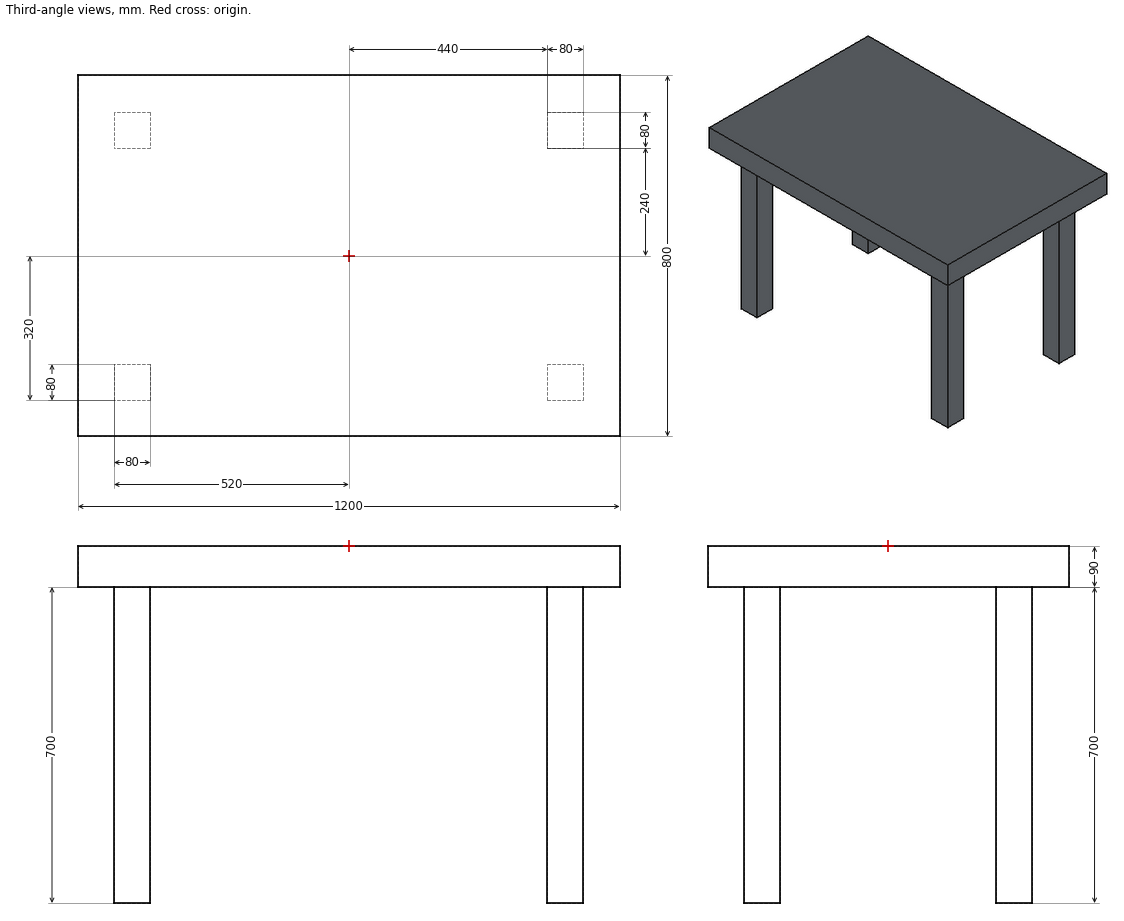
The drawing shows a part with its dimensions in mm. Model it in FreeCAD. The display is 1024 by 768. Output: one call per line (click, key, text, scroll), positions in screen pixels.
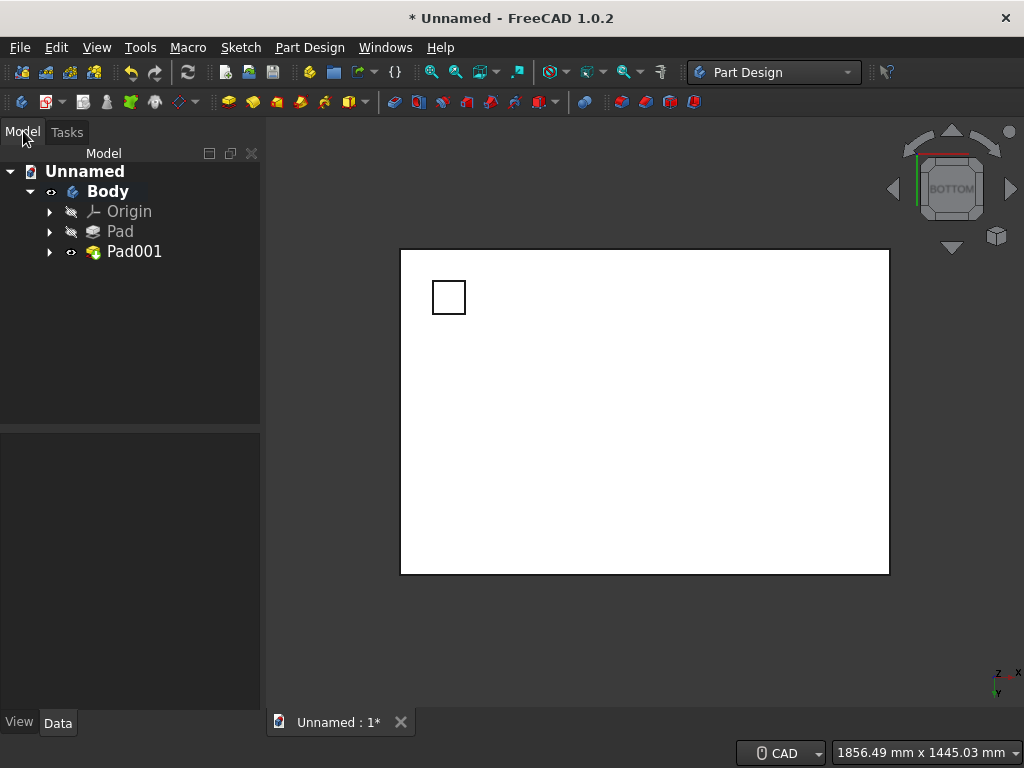
click(116, 252)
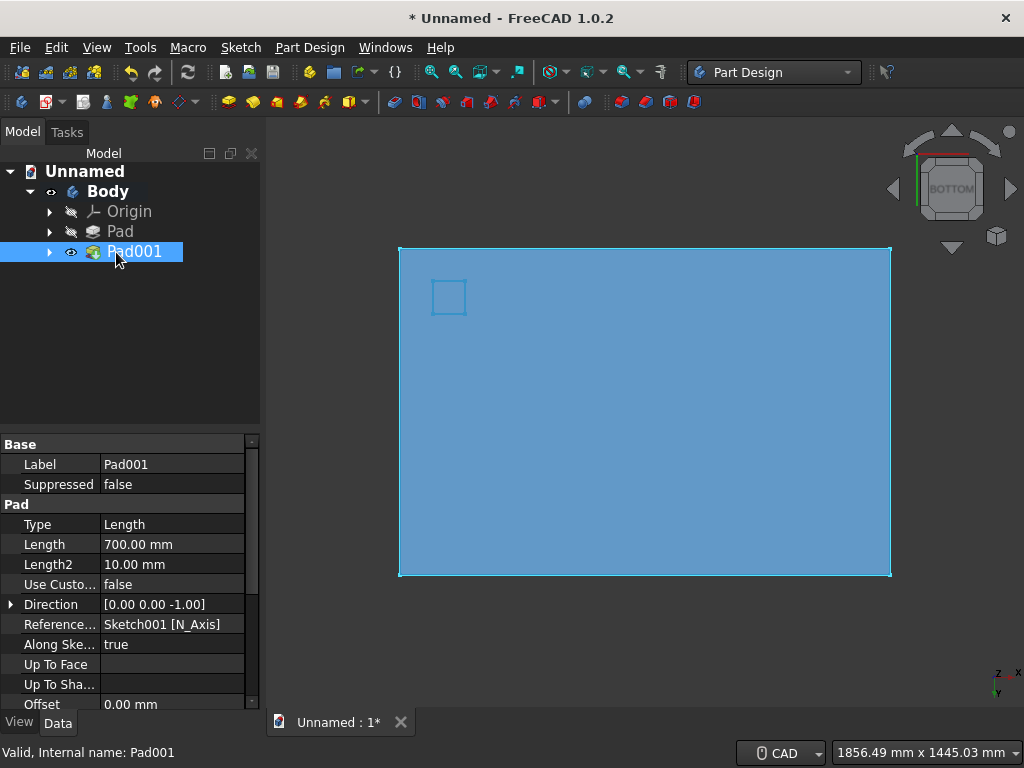
click(22, 72)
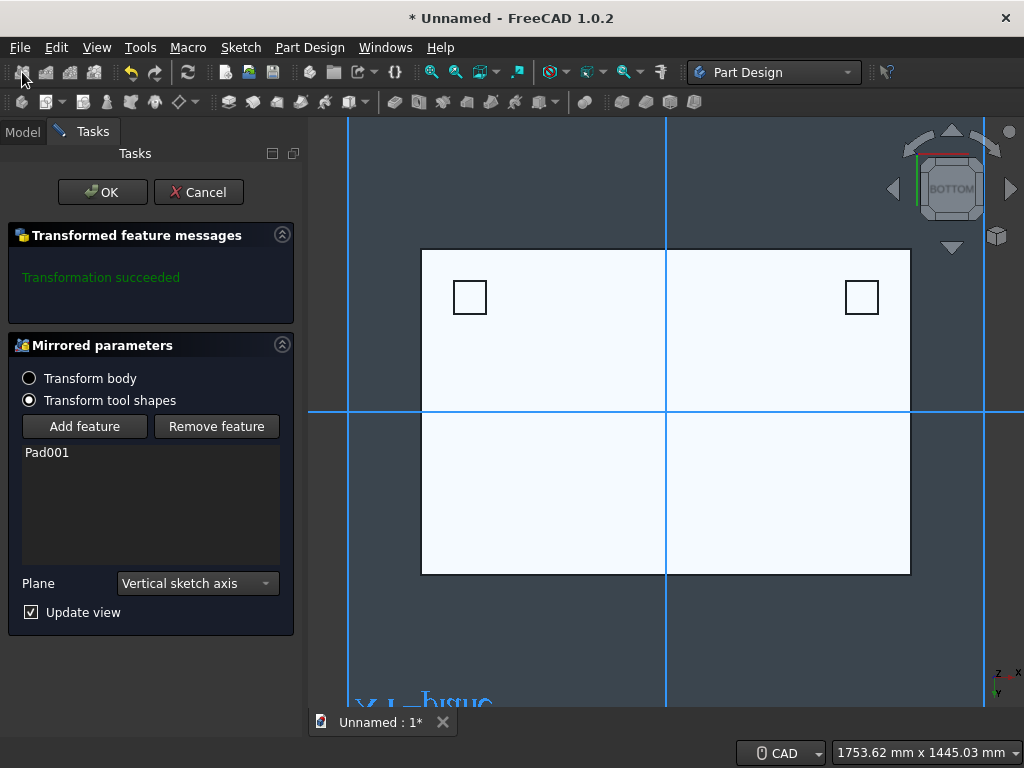
click(198, 584)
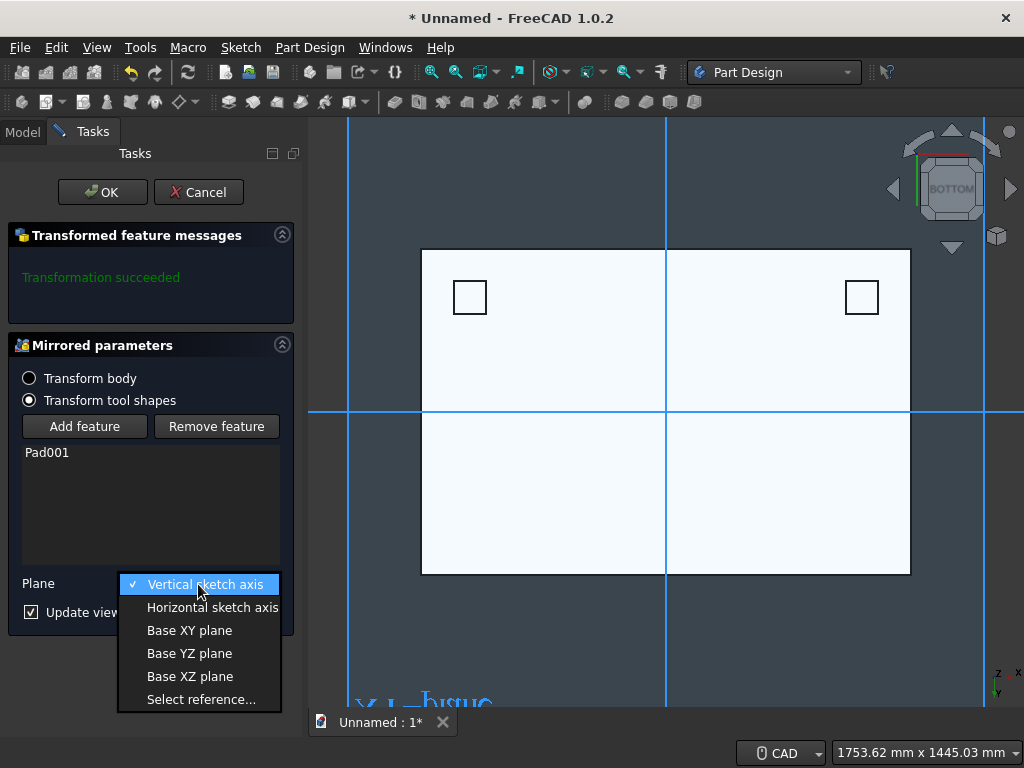
click(198, 676)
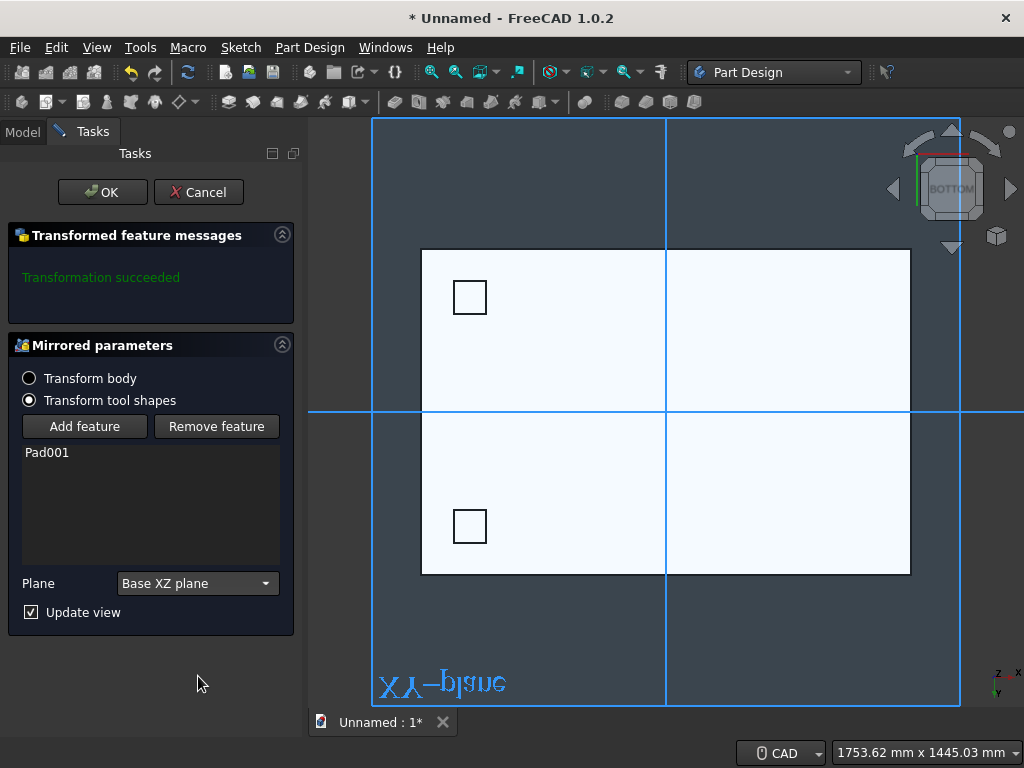
click(103, 192)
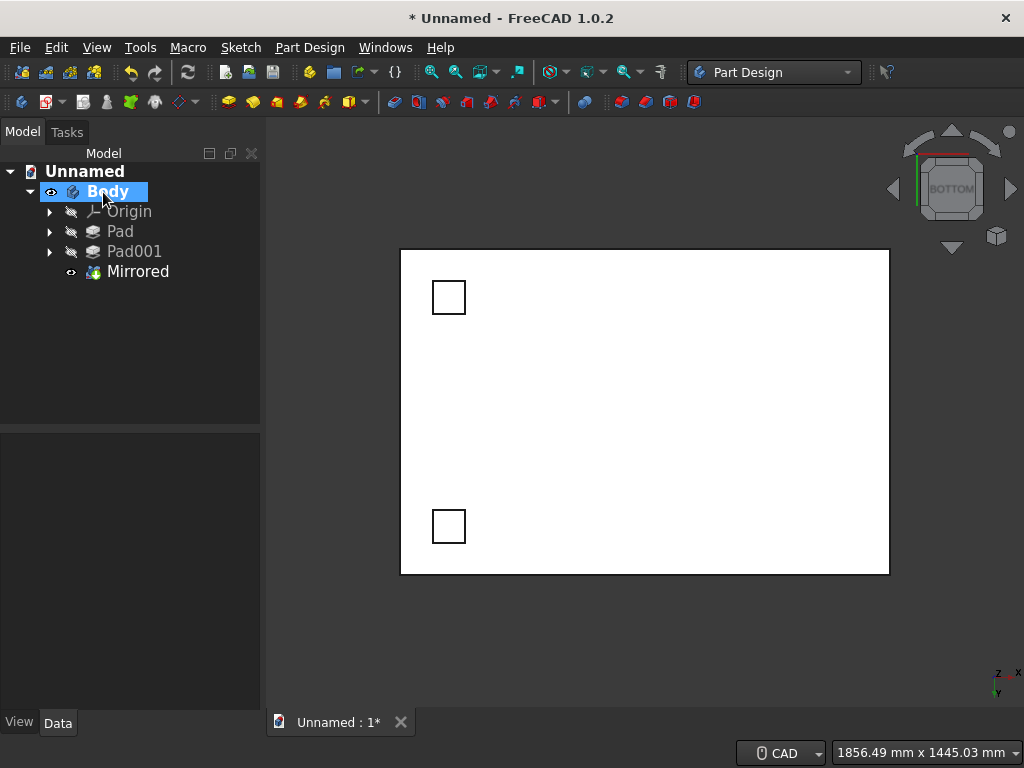
click(116, 252)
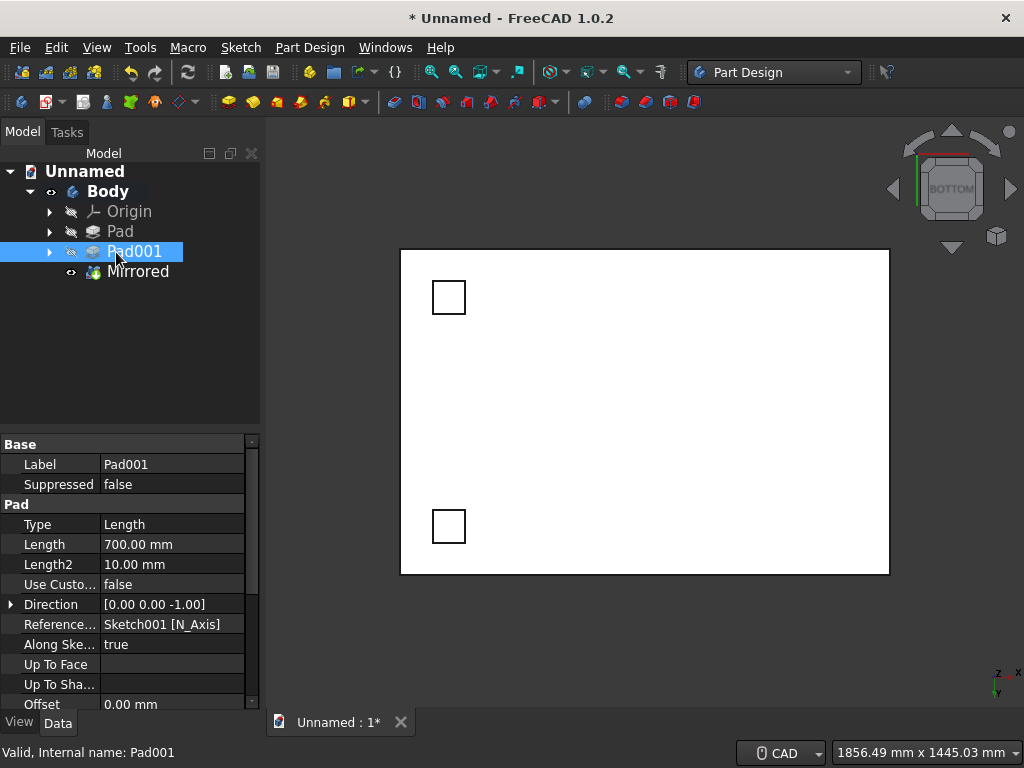
click(22, 72)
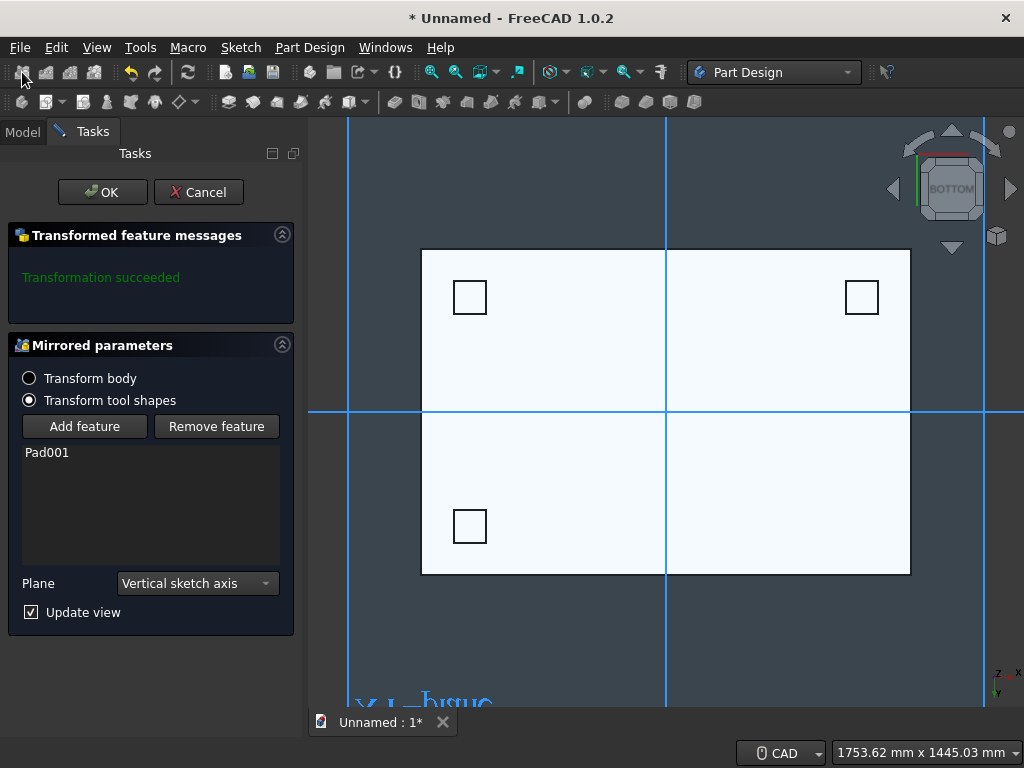
click(198, 584)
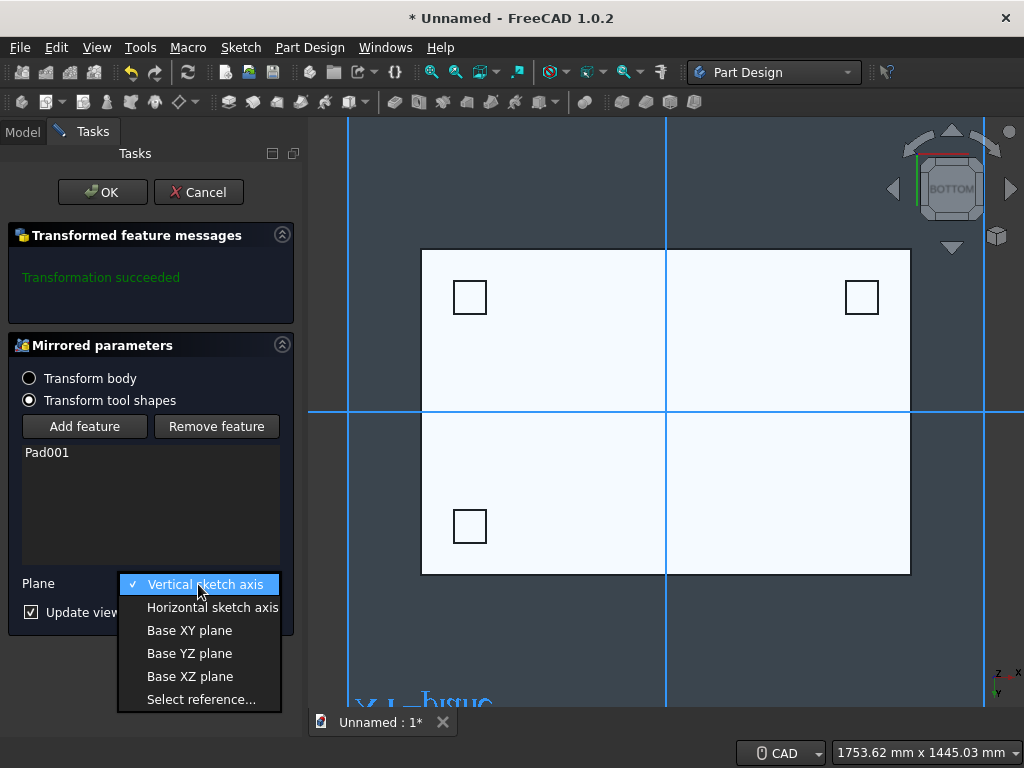
click(198, 654)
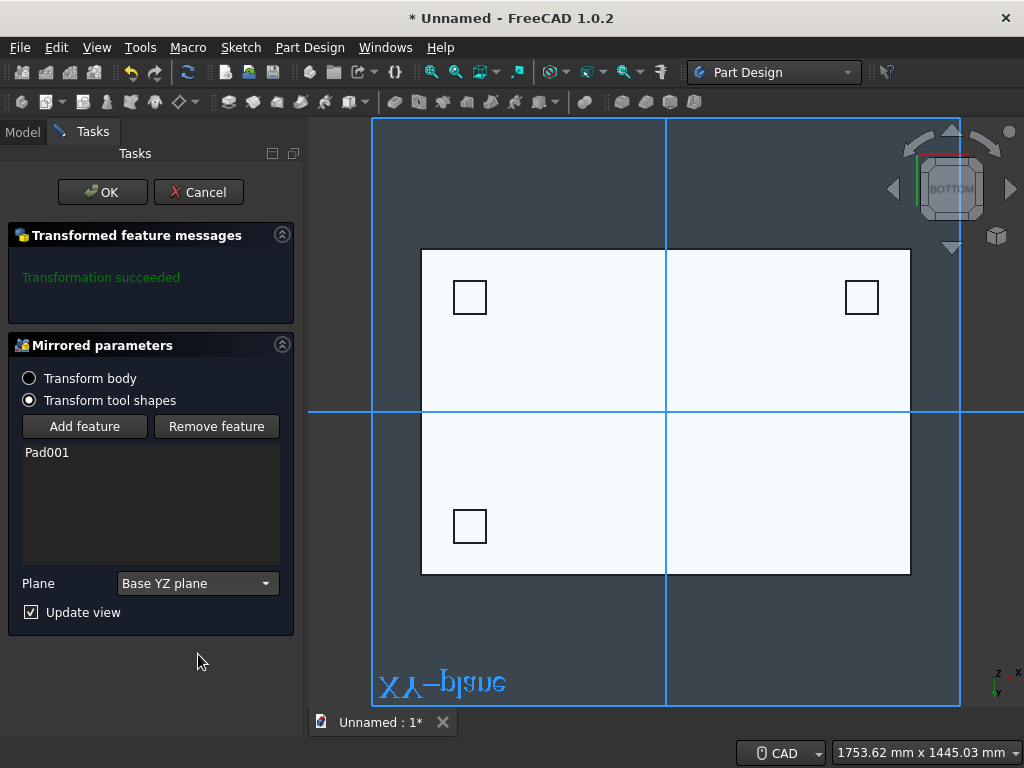
click(103, 192)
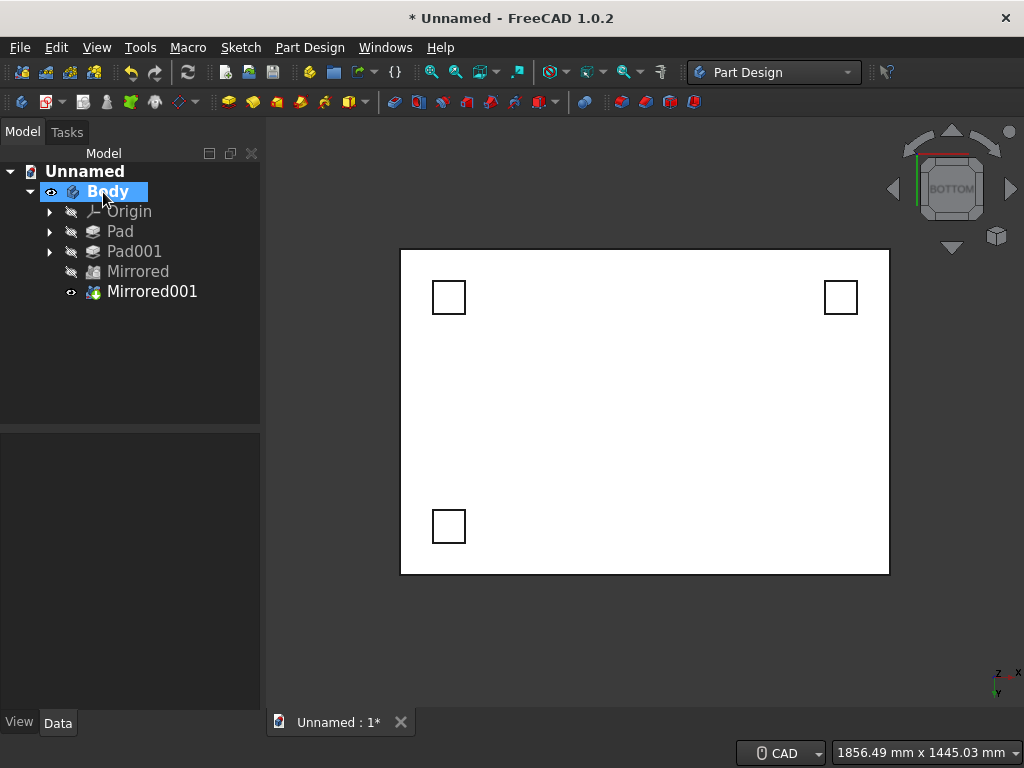
click(645, 411)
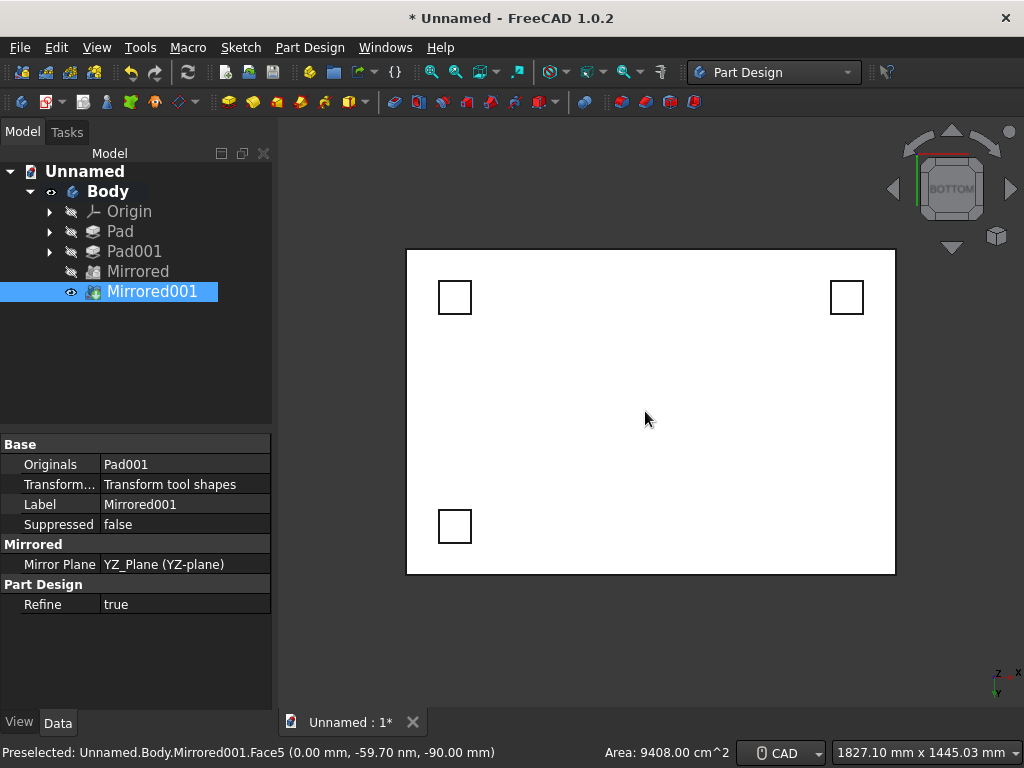
click(46, 102)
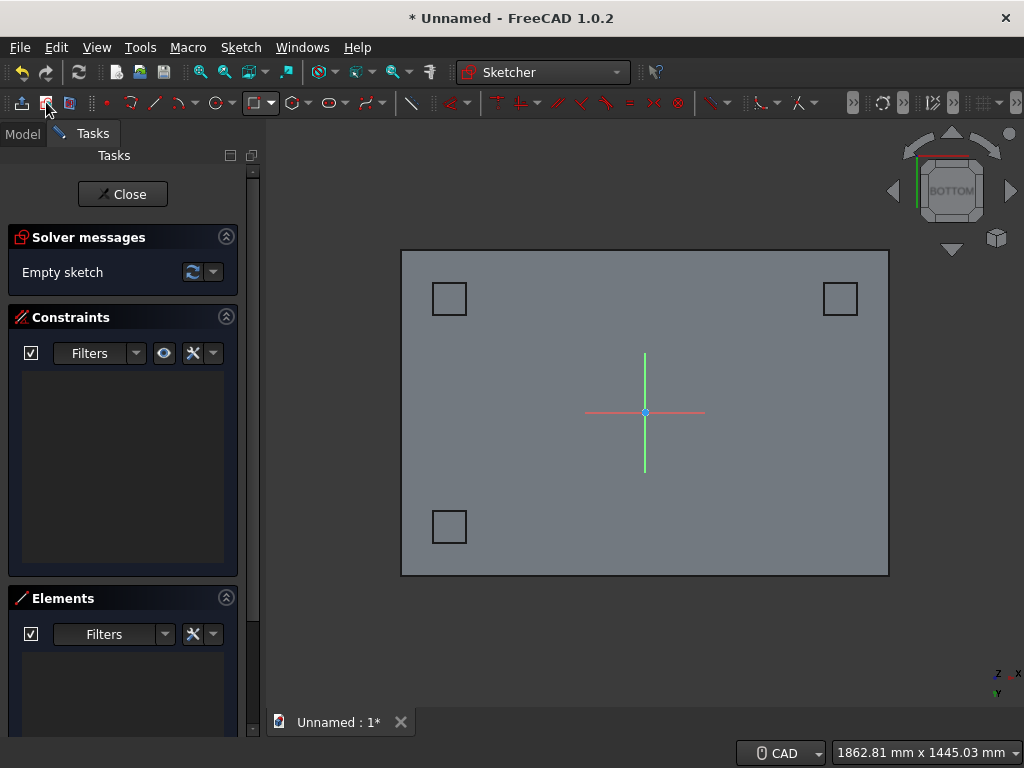
key(q)
key(s)